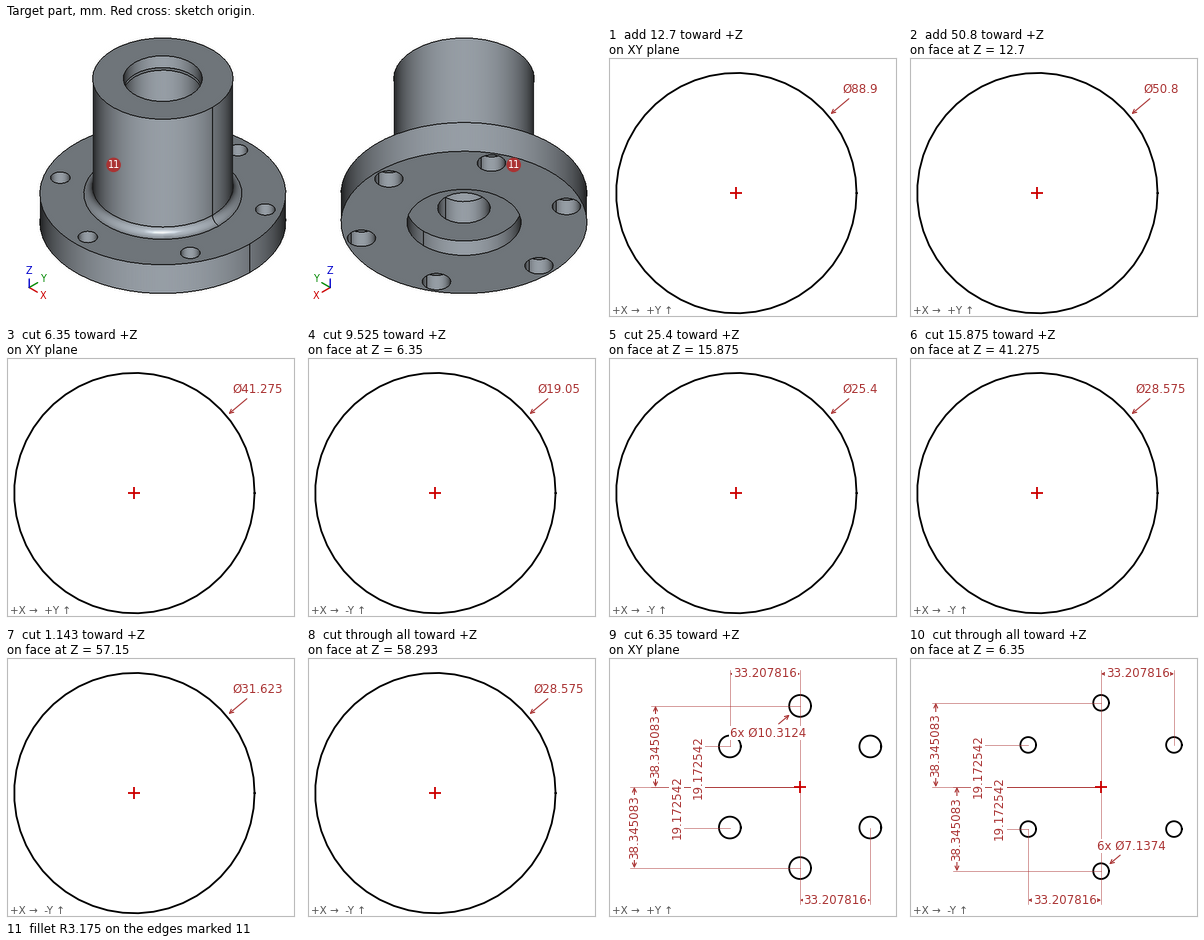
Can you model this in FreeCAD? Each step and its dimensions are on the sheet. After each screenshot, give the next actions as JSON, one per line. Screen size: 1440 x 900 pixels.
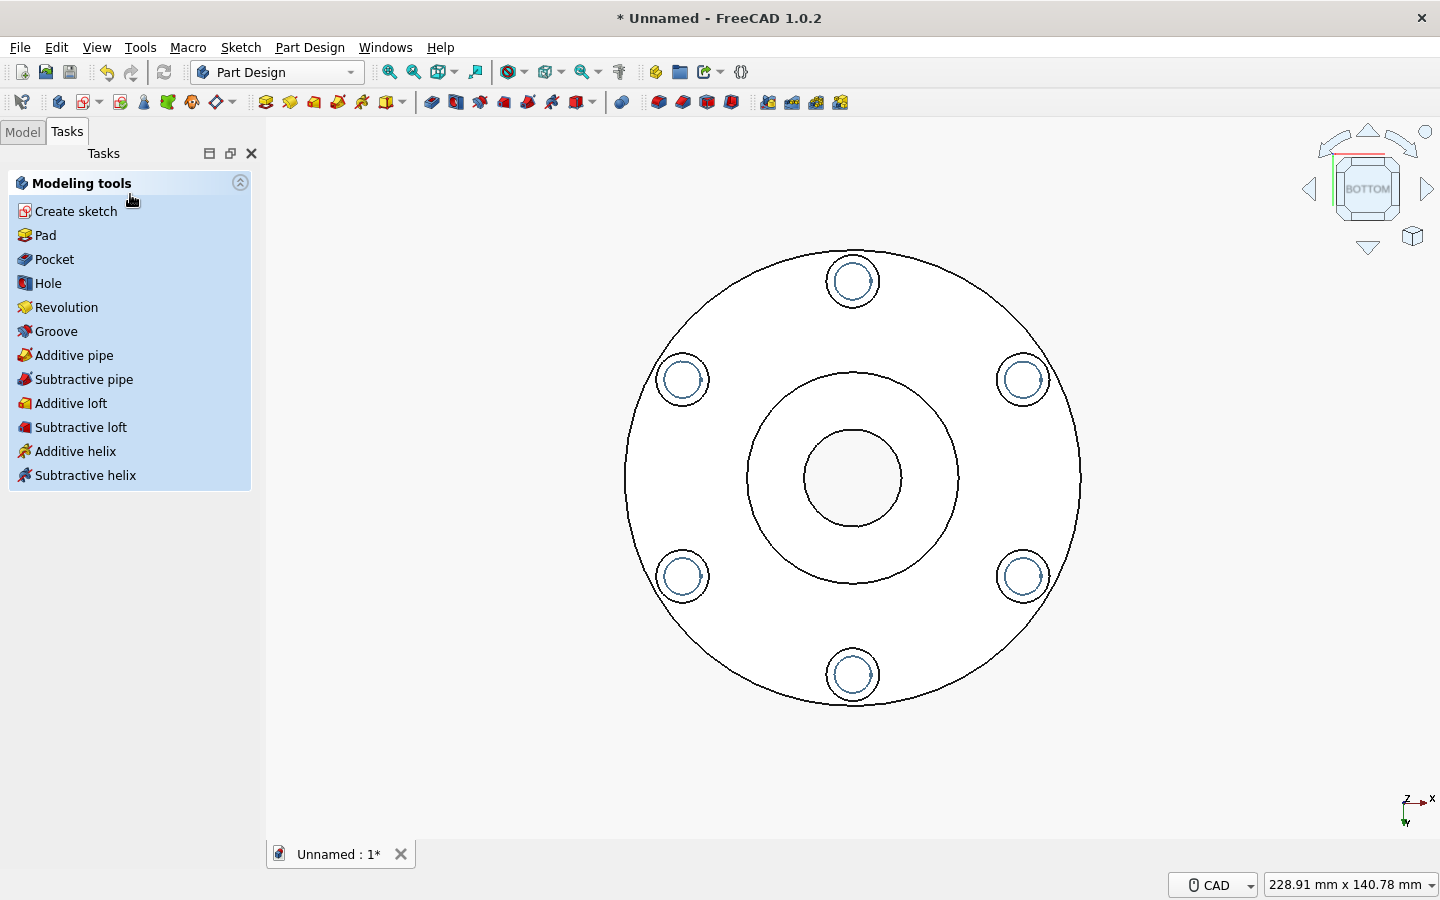
{"action": "left_click", "coordinate": [432, 102]}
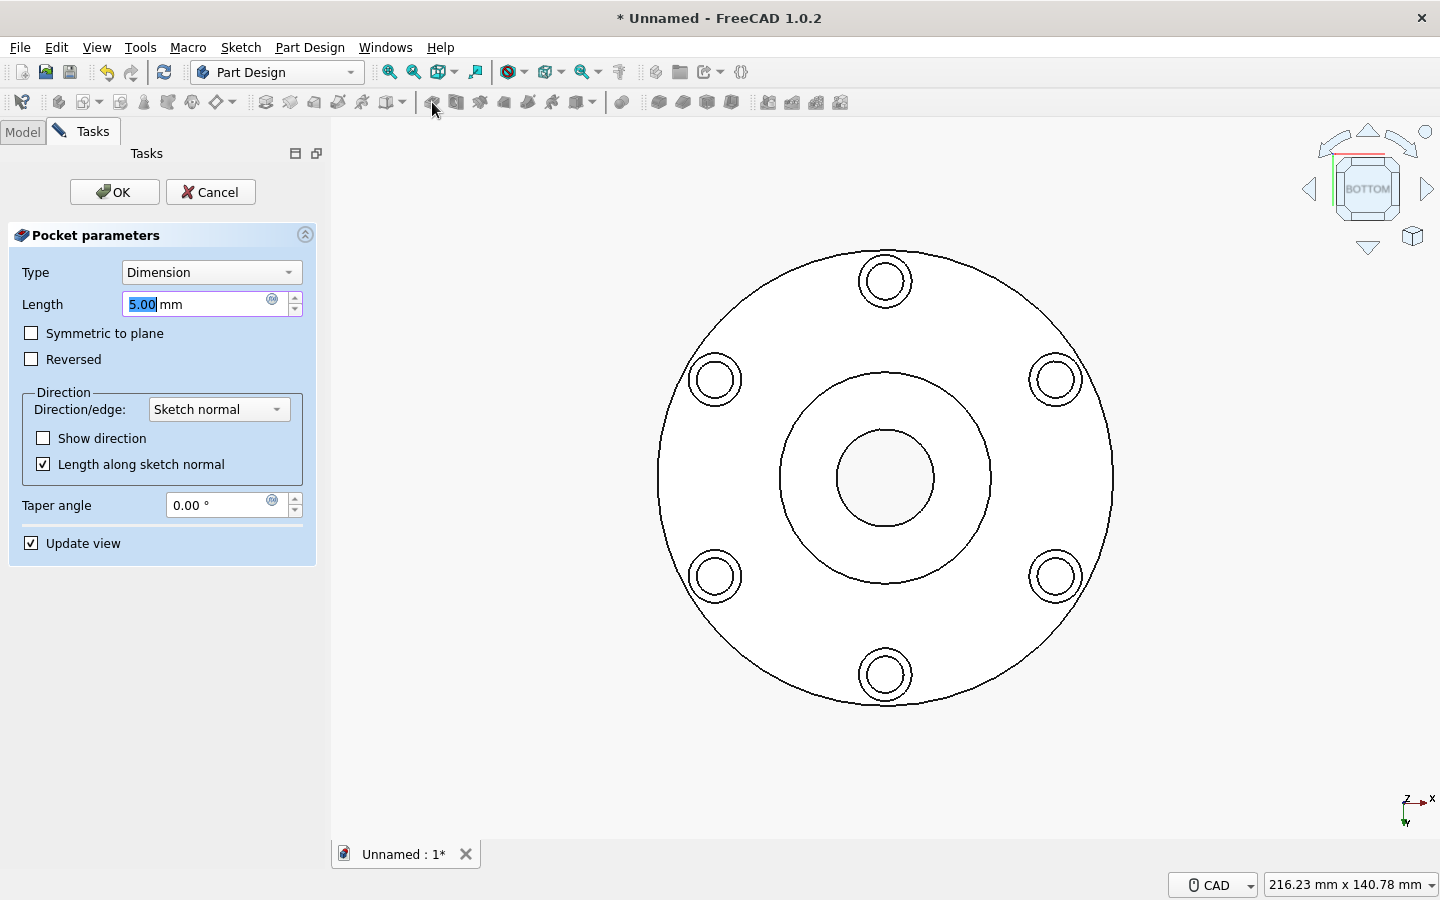
{"action": "left_click", "coordinate": [212, 272]}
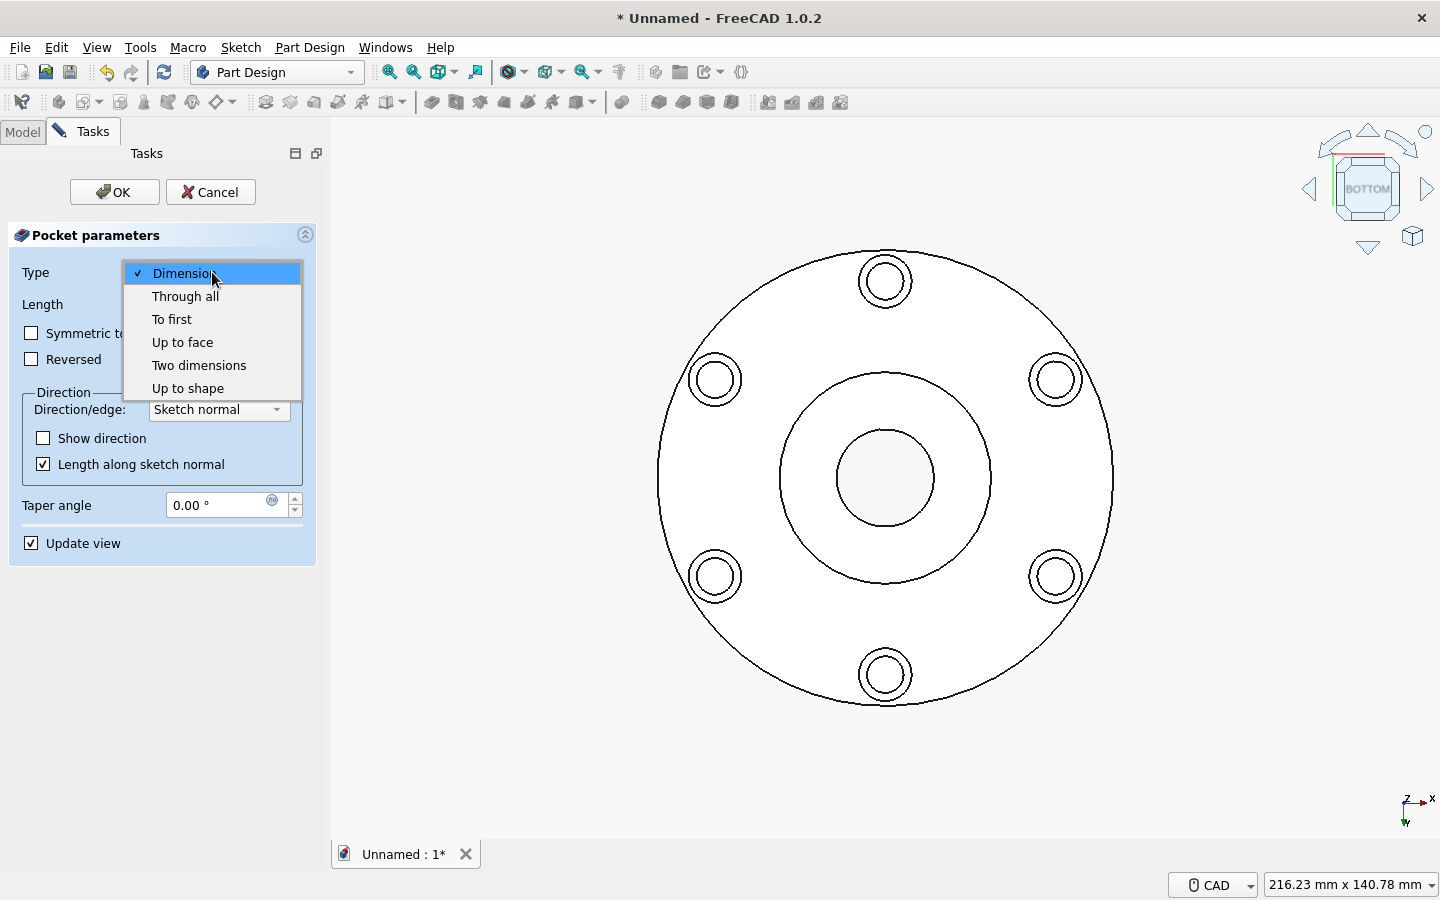
{"action": "left_click", "coordinate": [212, 296]}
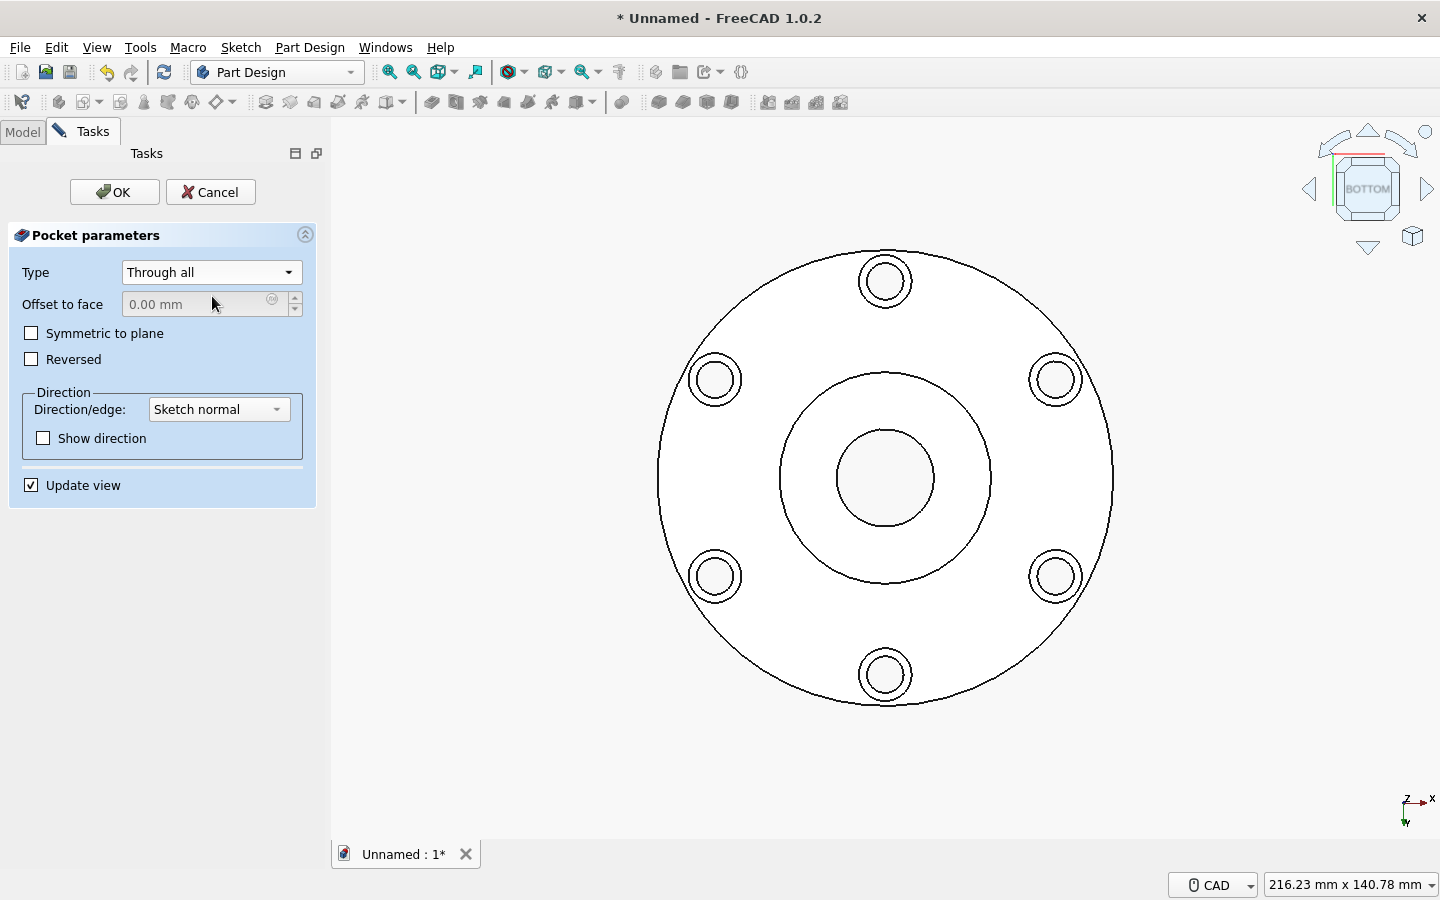
{"action": "left_click", "coordinate": [115, 192]}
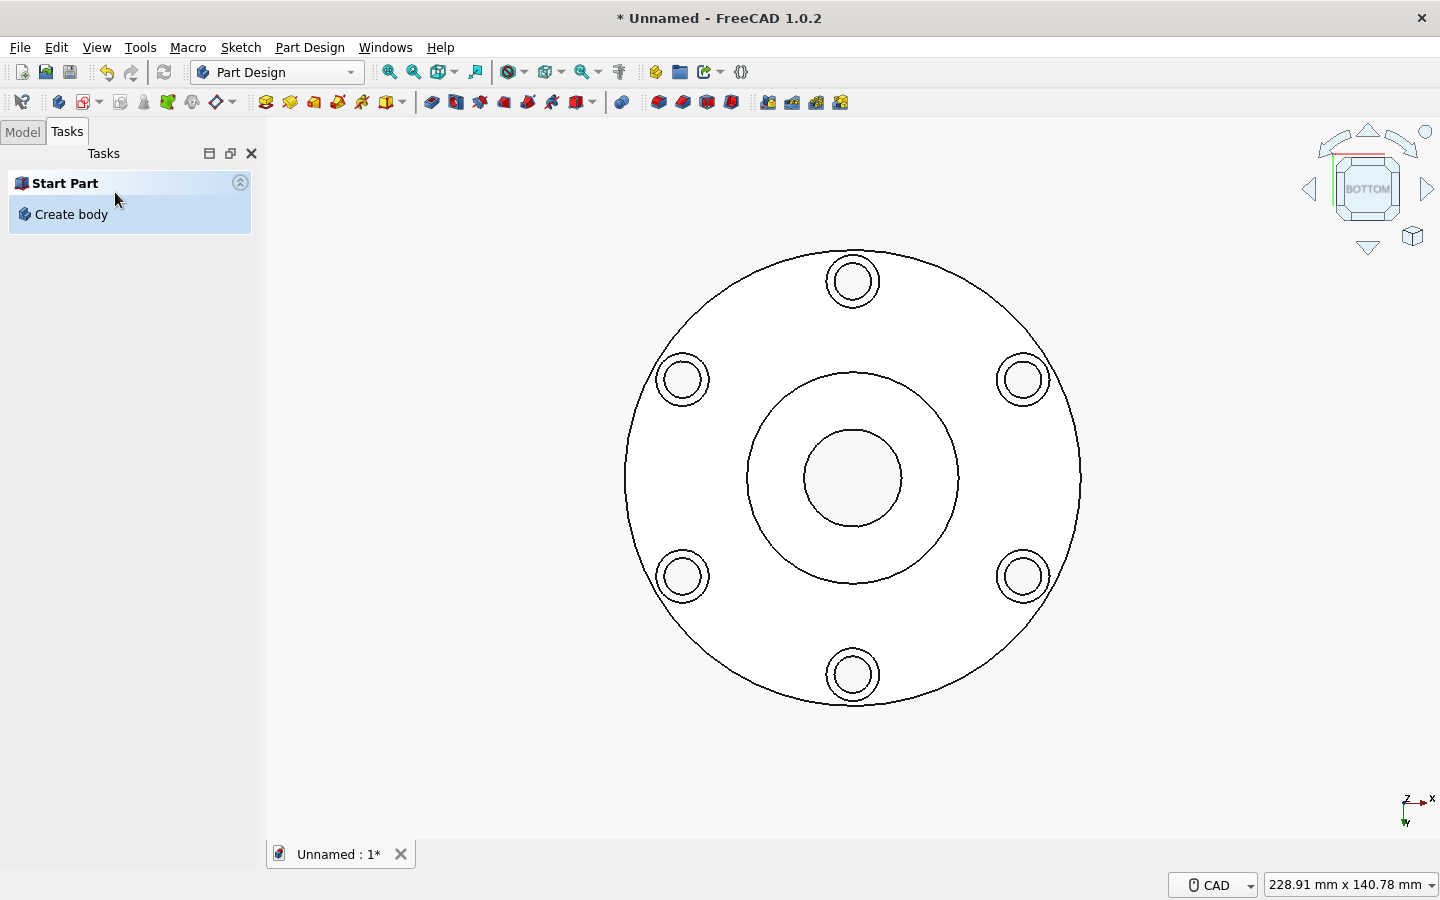
{"action": "key", "text": "0"}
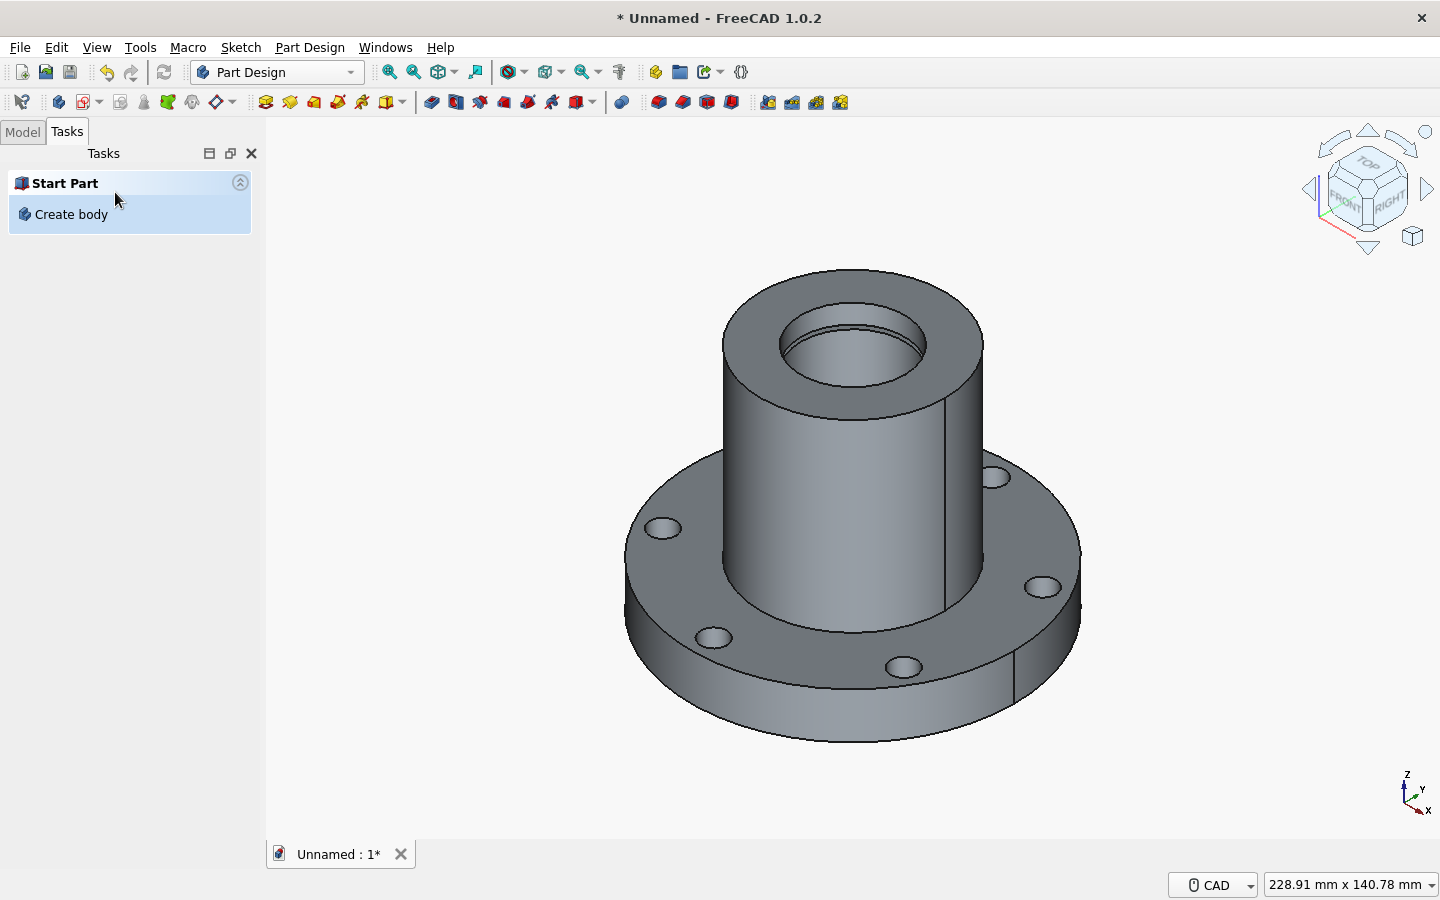
{"action": "key", "text": "2"}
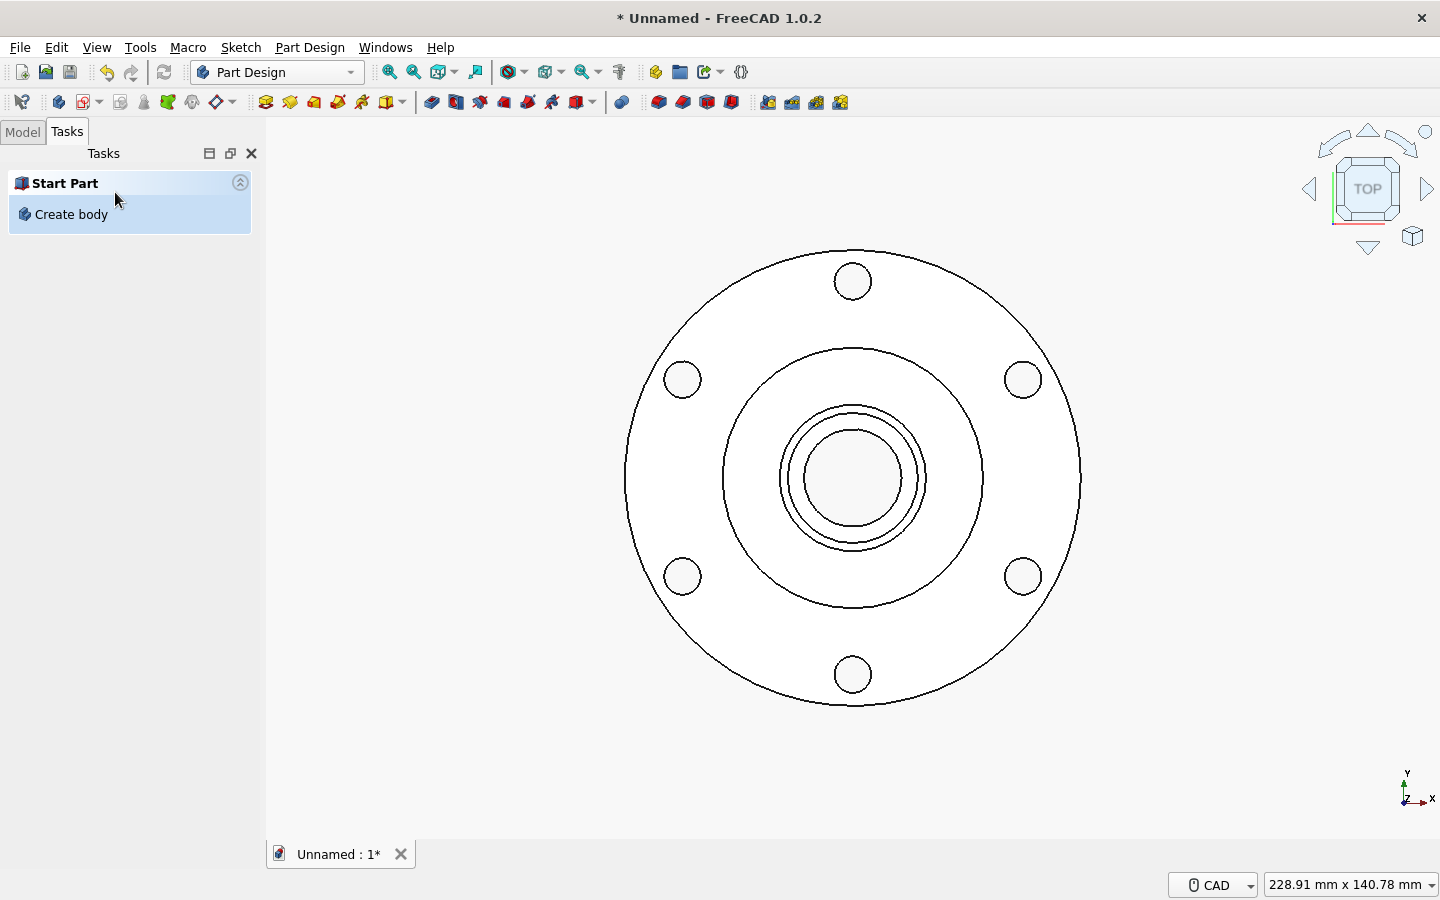
{"action": "key", "text": "1"}